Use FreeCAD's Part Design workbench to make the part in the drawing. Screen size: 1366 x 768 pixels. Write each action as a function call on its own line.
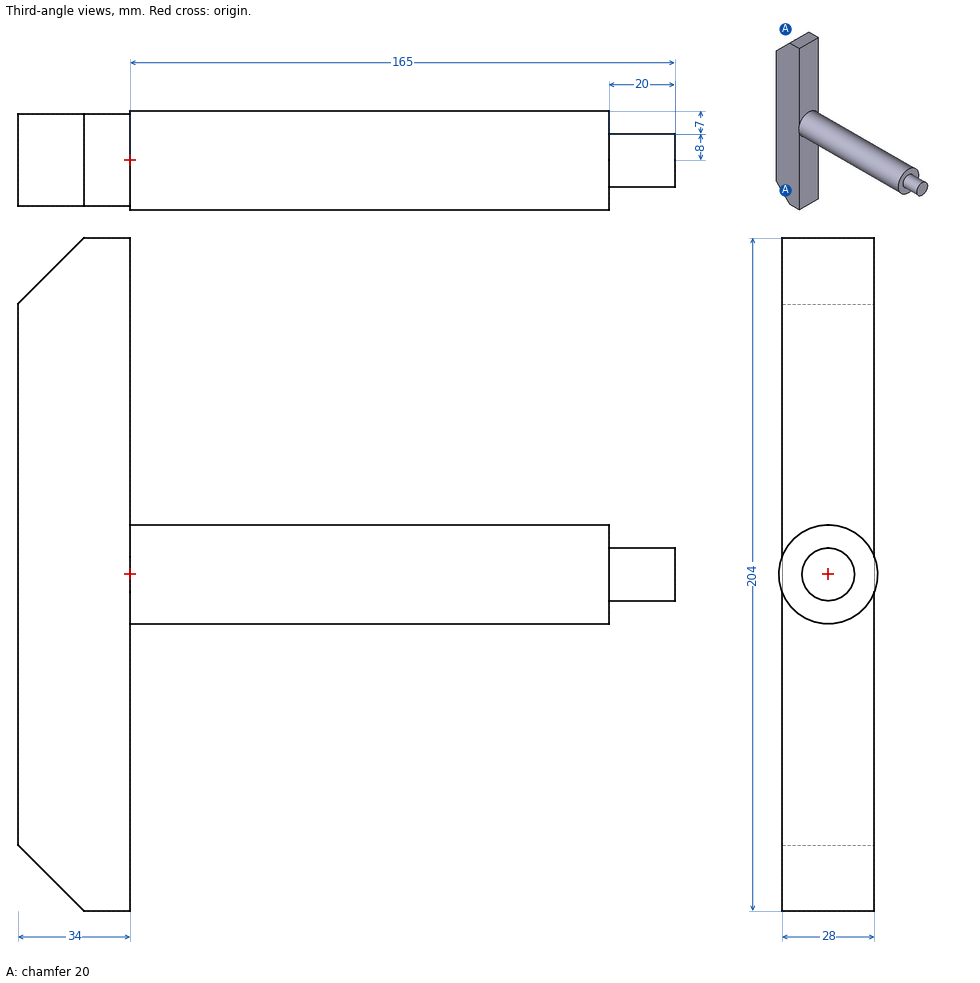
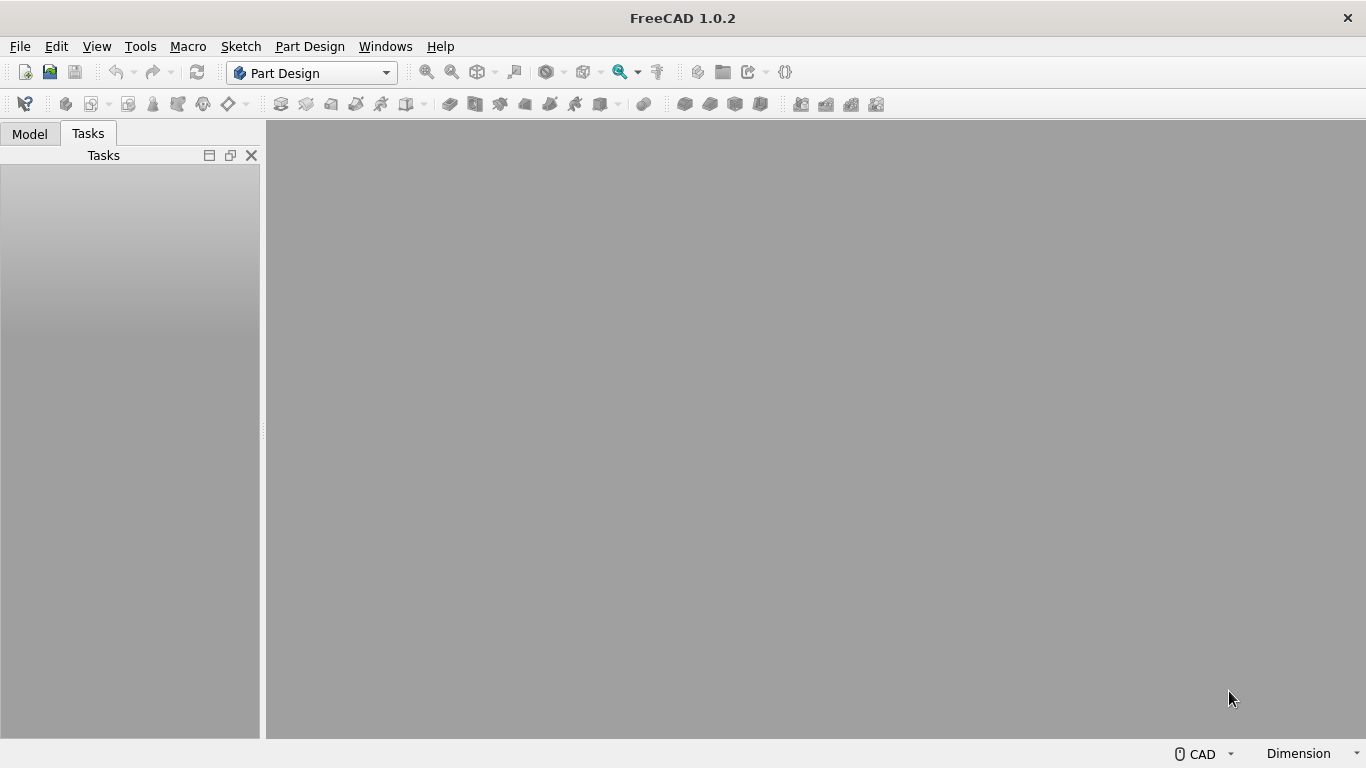
click(25, 72)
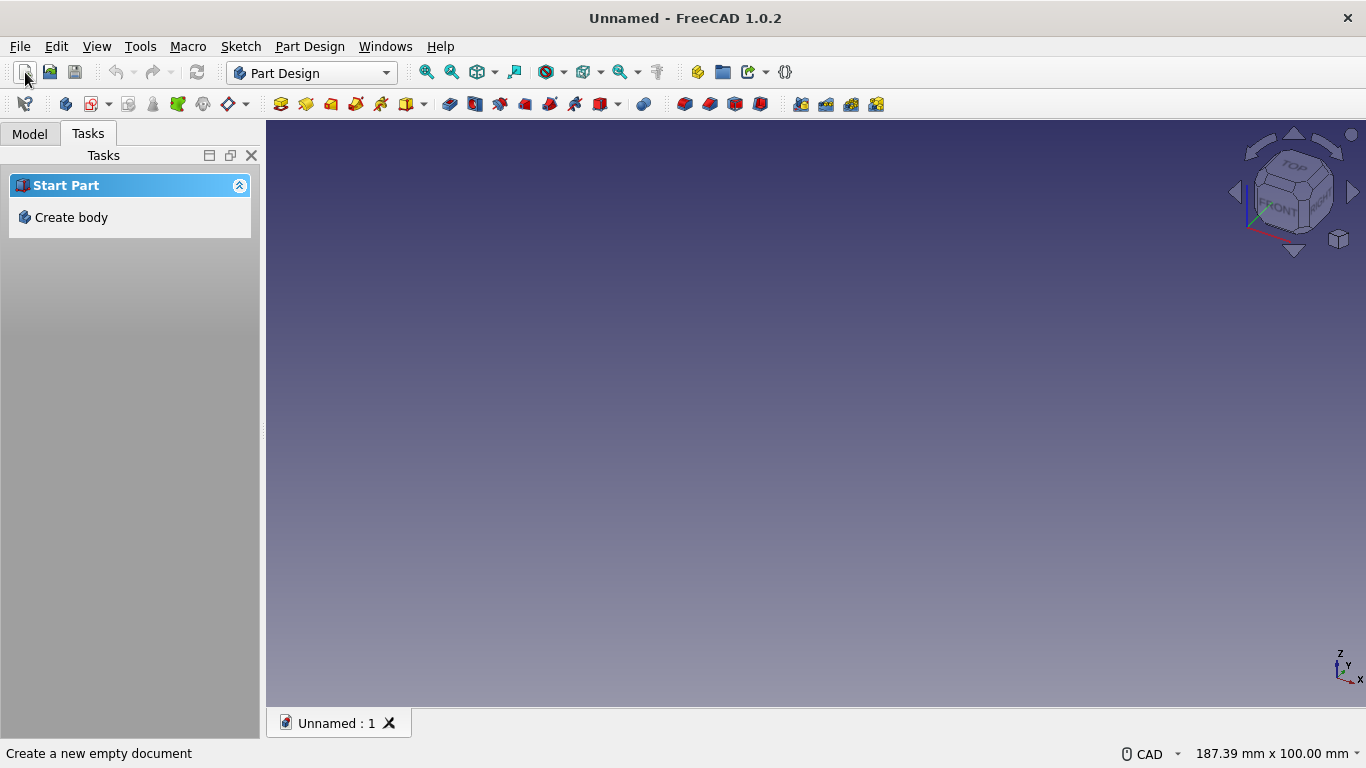
click(90, 104)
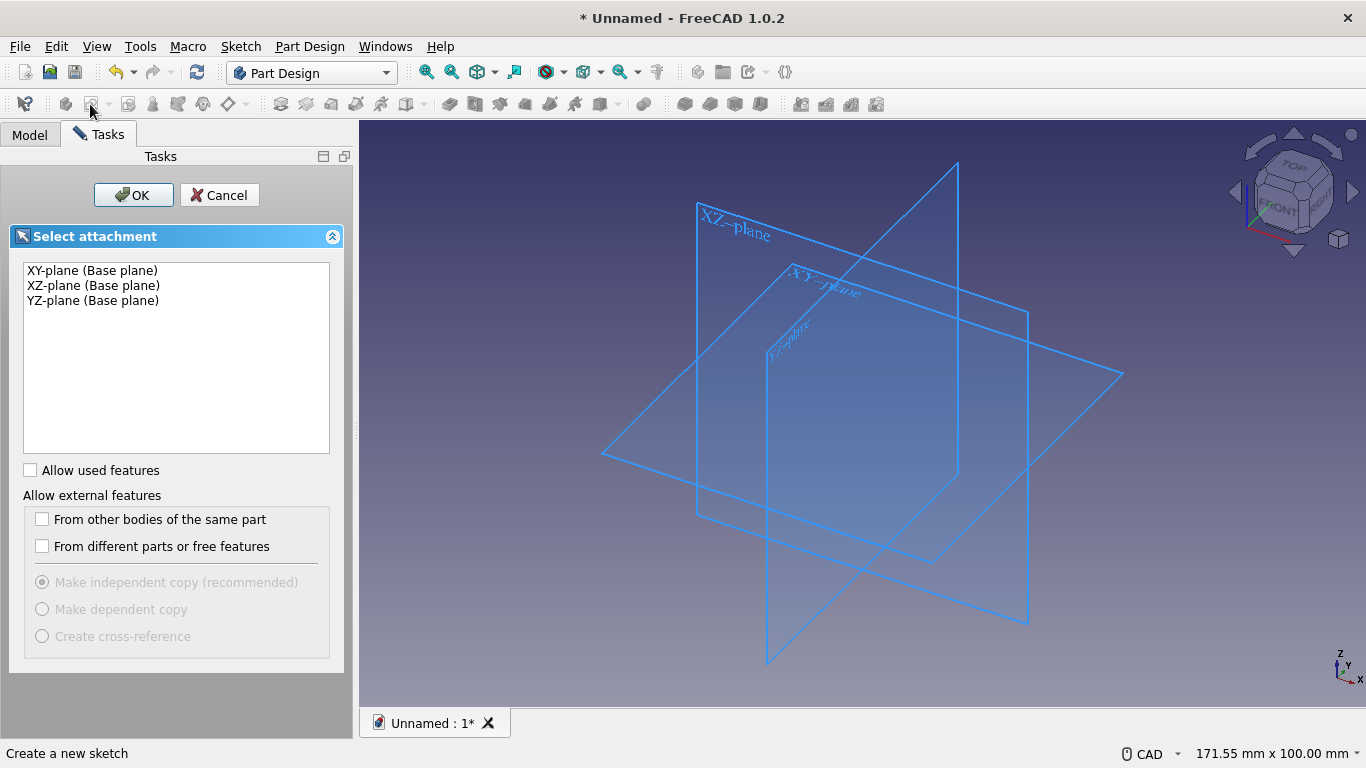
click(84, 270)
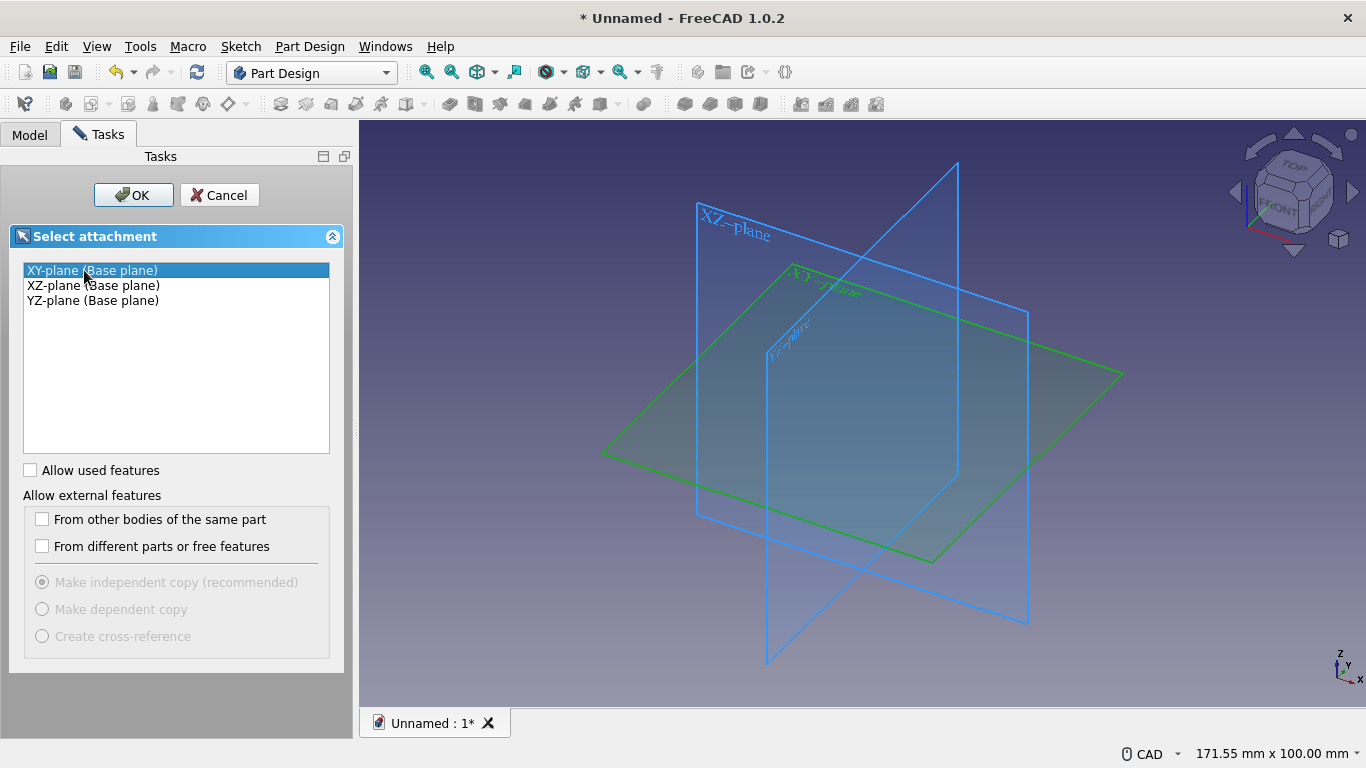
click(134, 195)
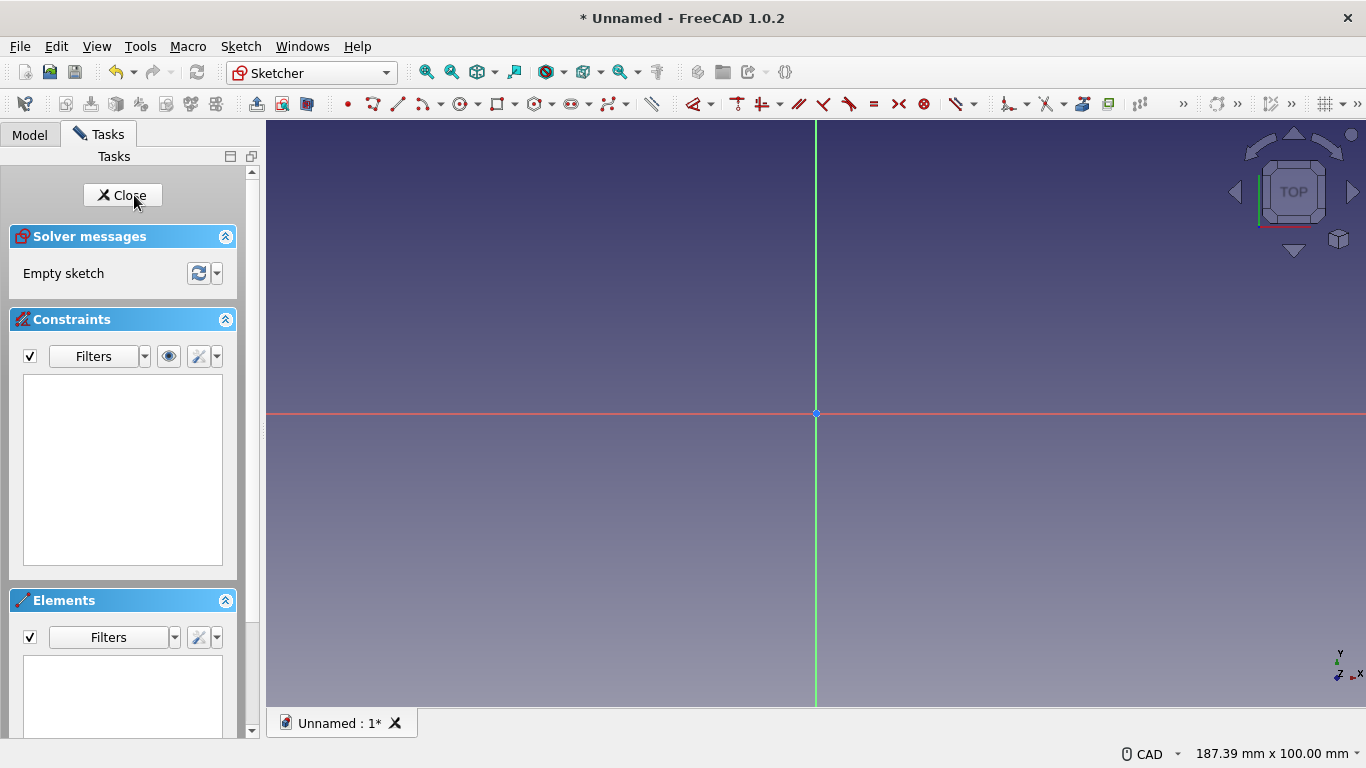
scroll(294, 467, down, 3)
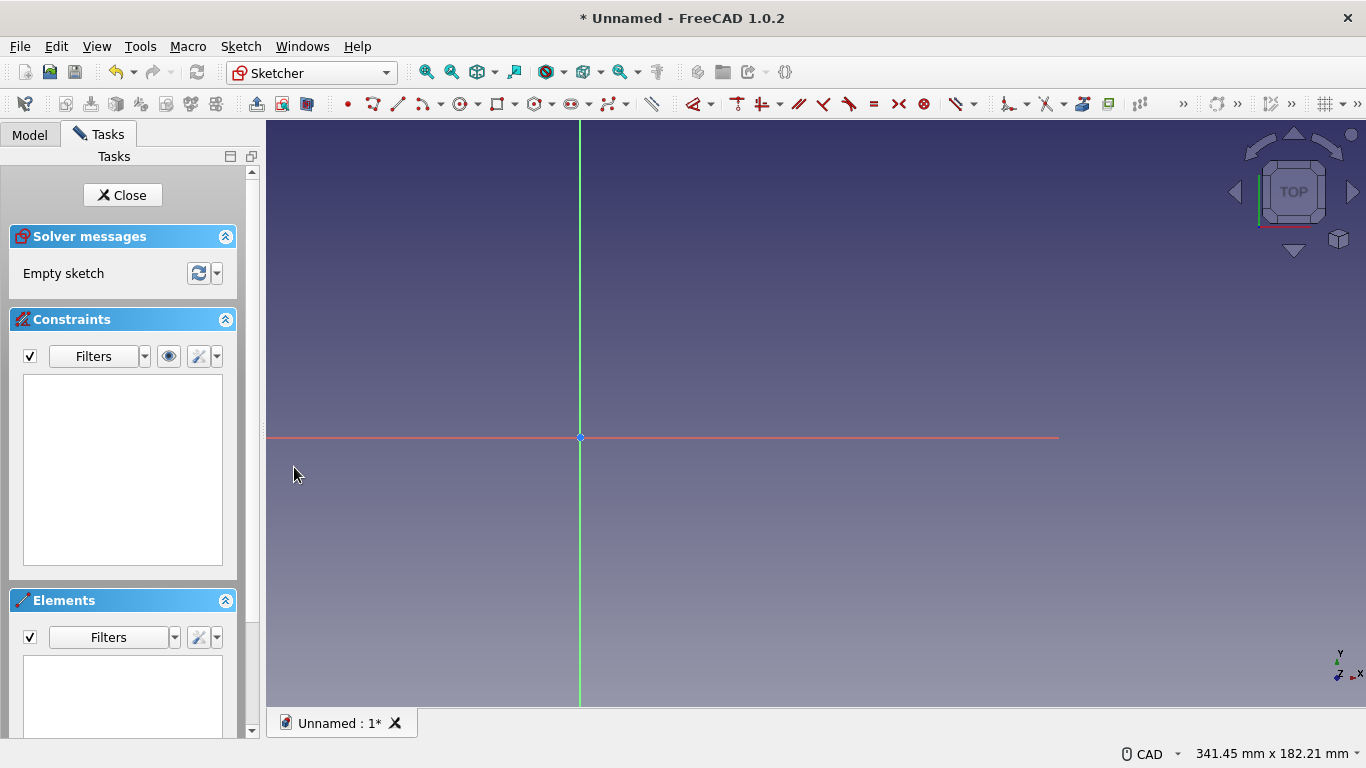
click(373, 104)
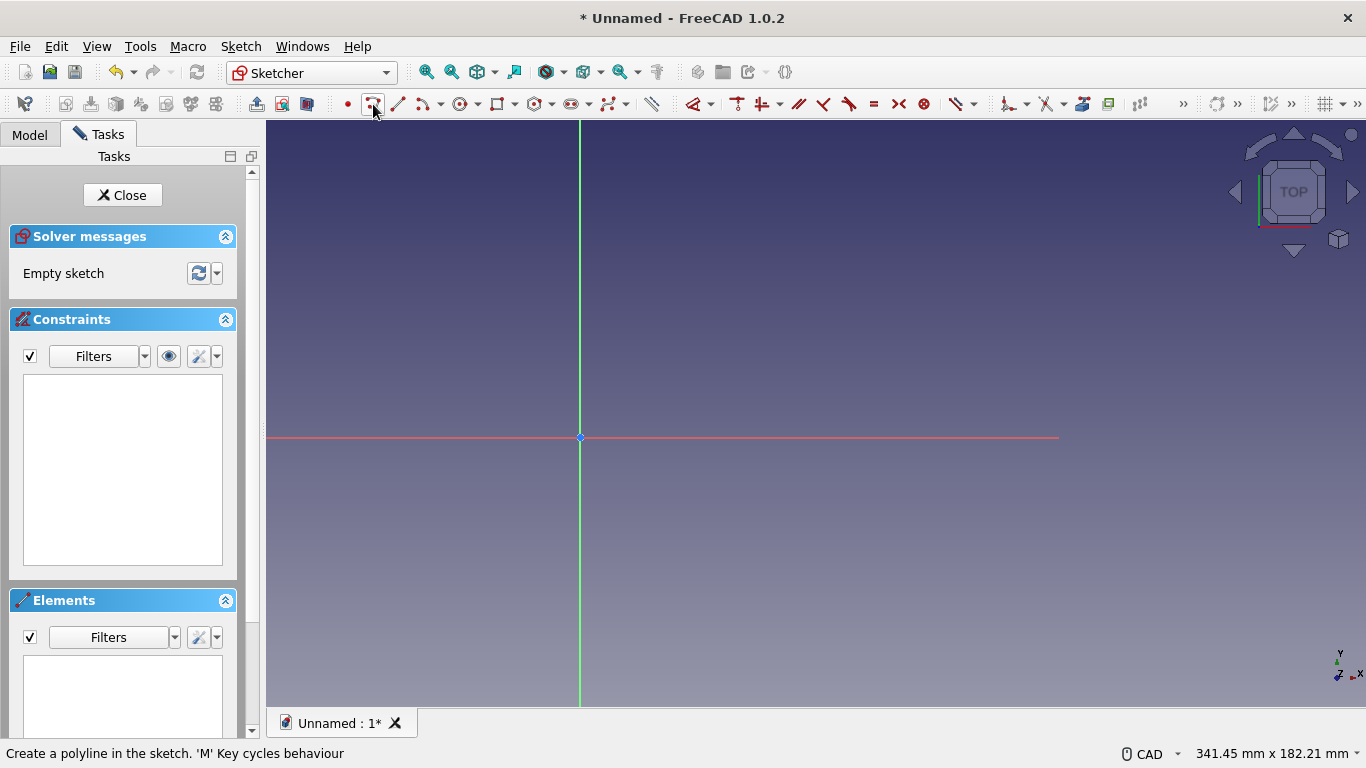
click(580, 438)
click(1112, 429)
click(1112, 412)
click(1048, 412)
click(1048, 390)
click(589, 390)
click(580, 438)
key(Escape)
key(Escape)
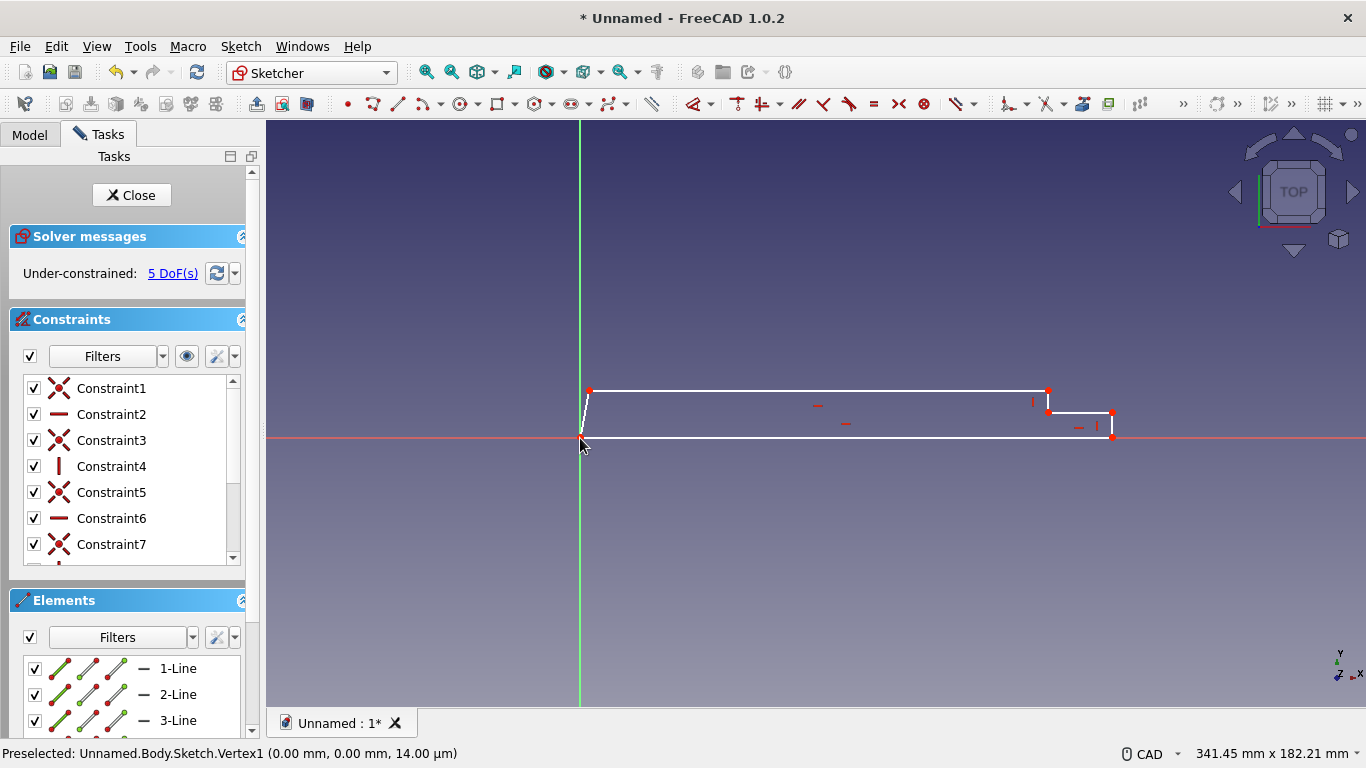
click(583, 424)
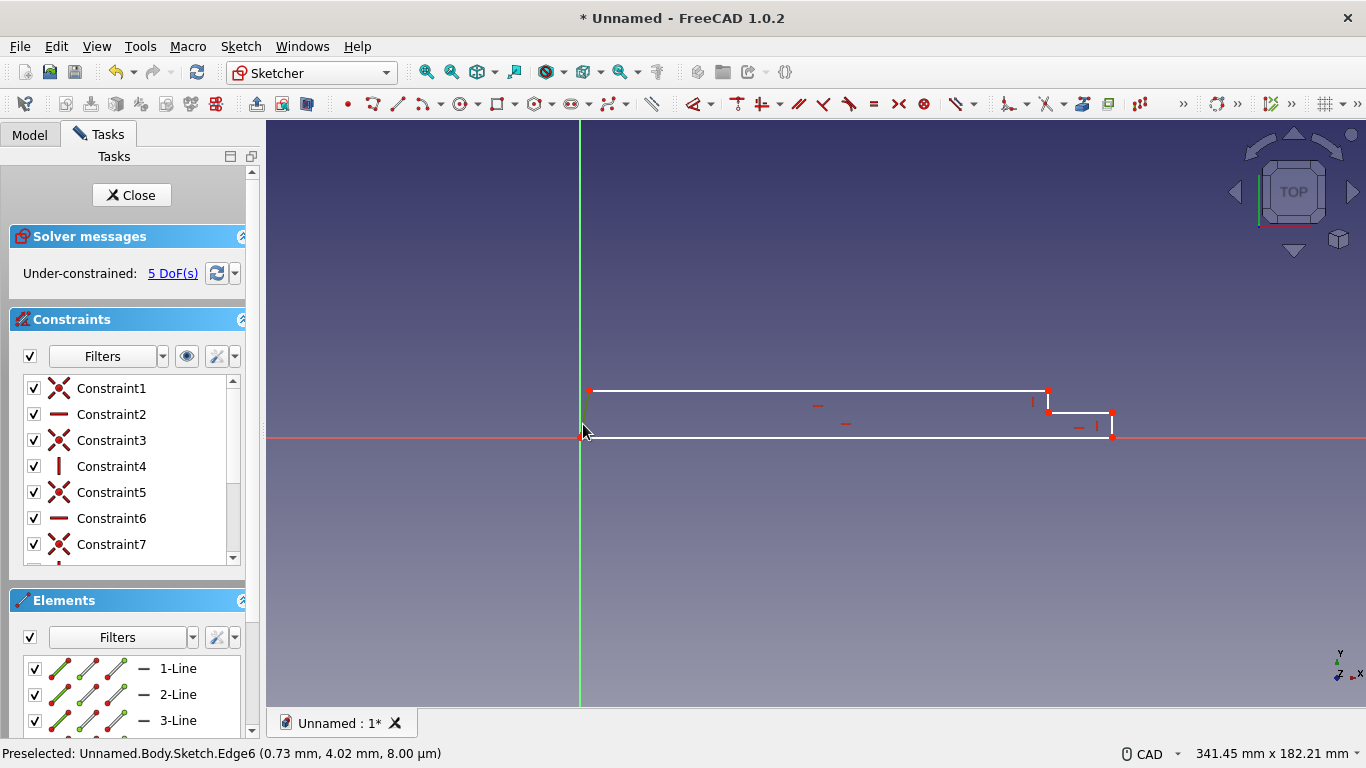
click(780, 104)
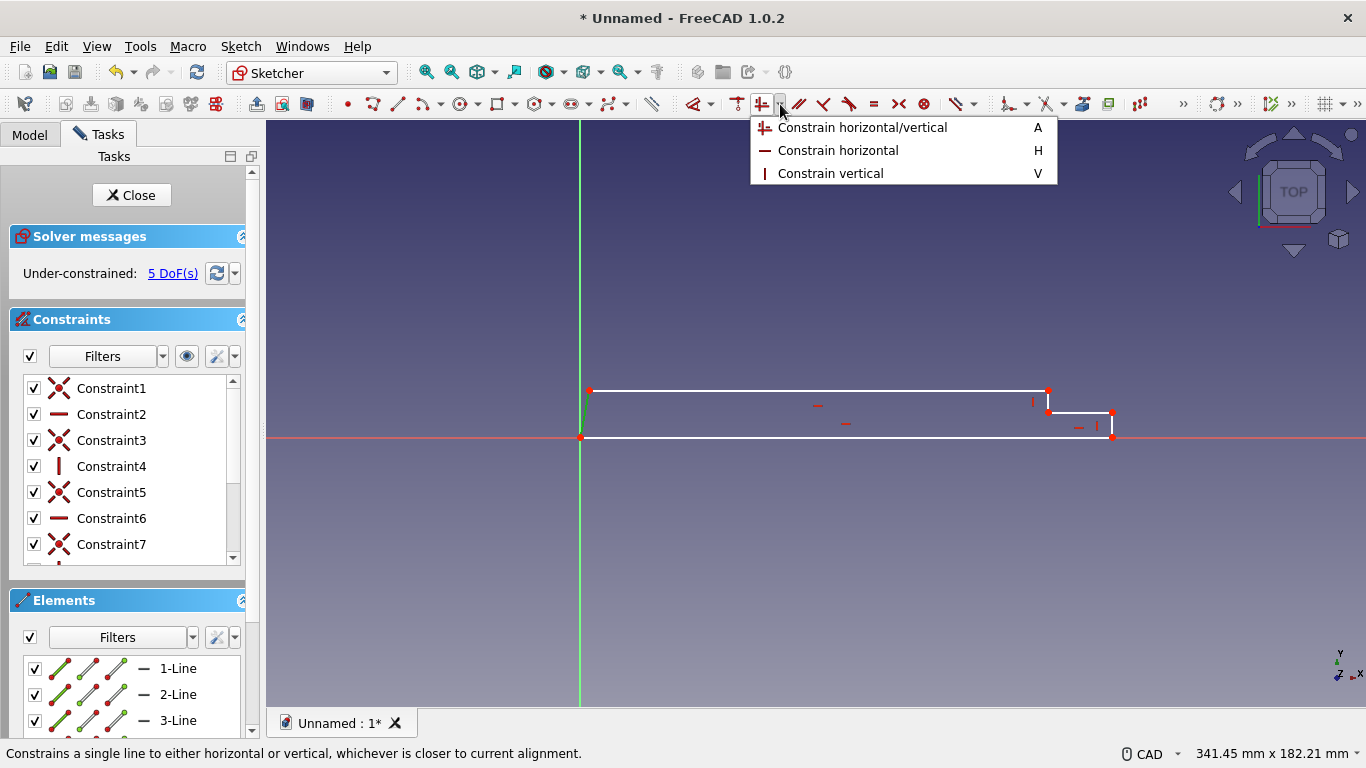
click(904, 174)